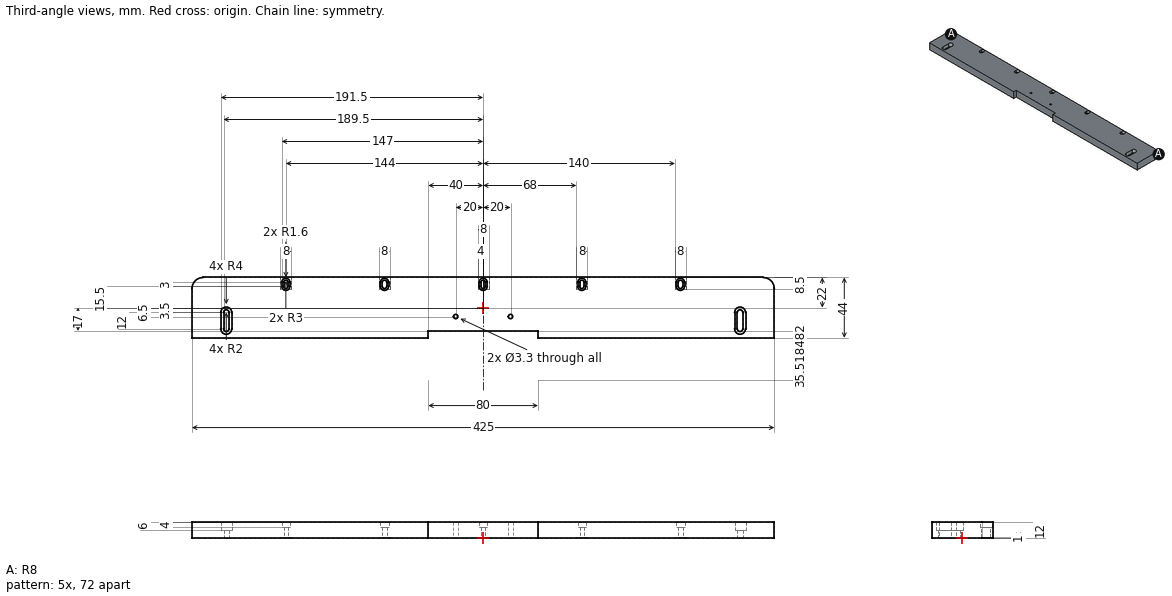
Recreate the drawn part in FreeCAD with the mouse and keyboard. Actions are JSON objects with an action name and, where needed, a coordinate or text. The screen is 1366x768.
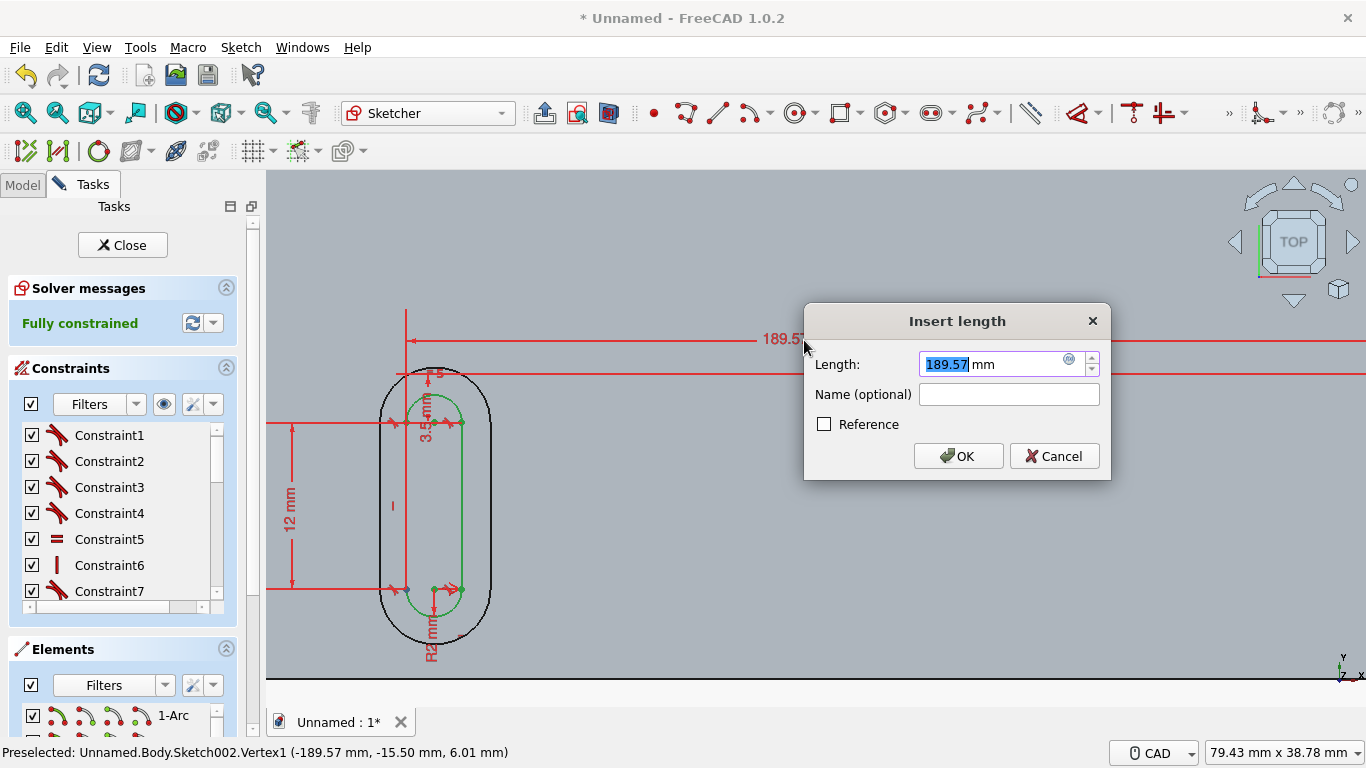
{"action": "type", "text": "189.5"}
{"action": "key", "text": "Return"}
{"action": "key", "text": "Escape"}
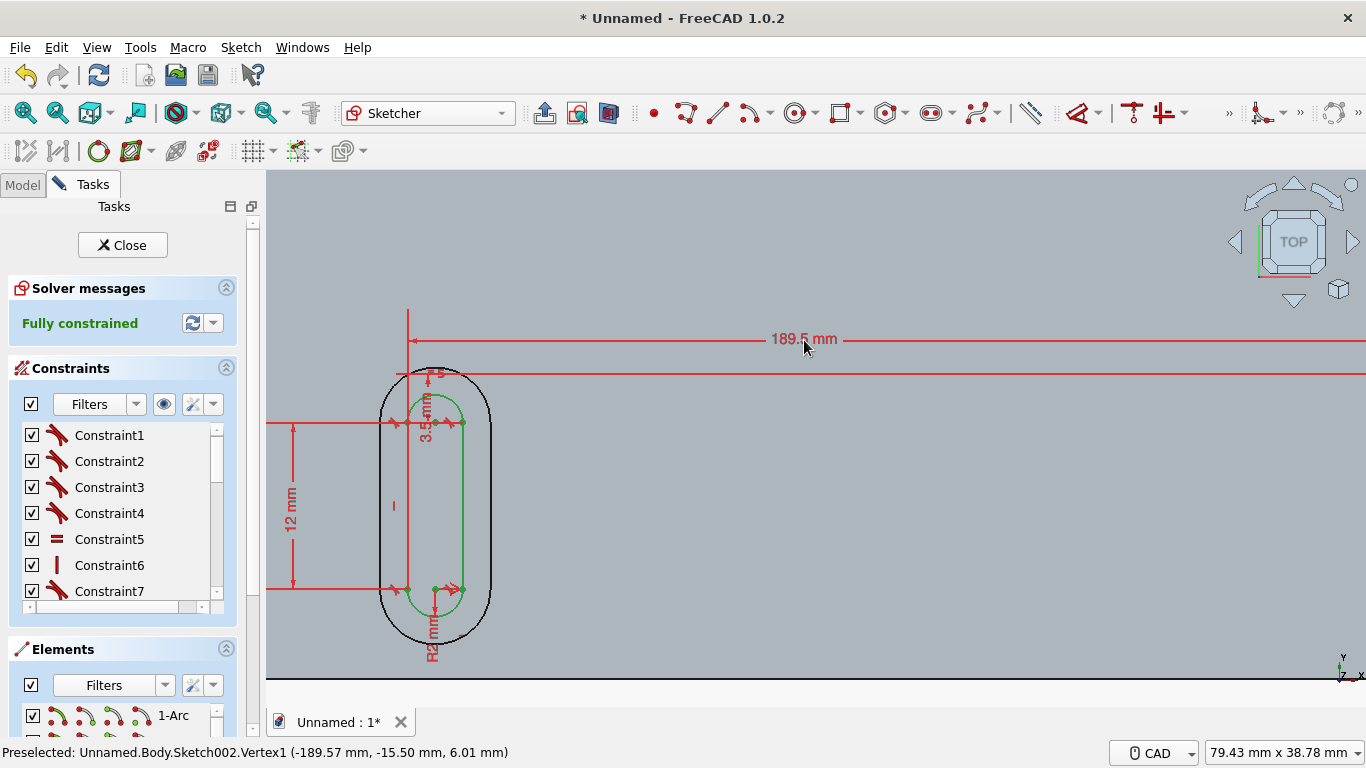
{"action": "left_click", "coordinate": [123, 245]}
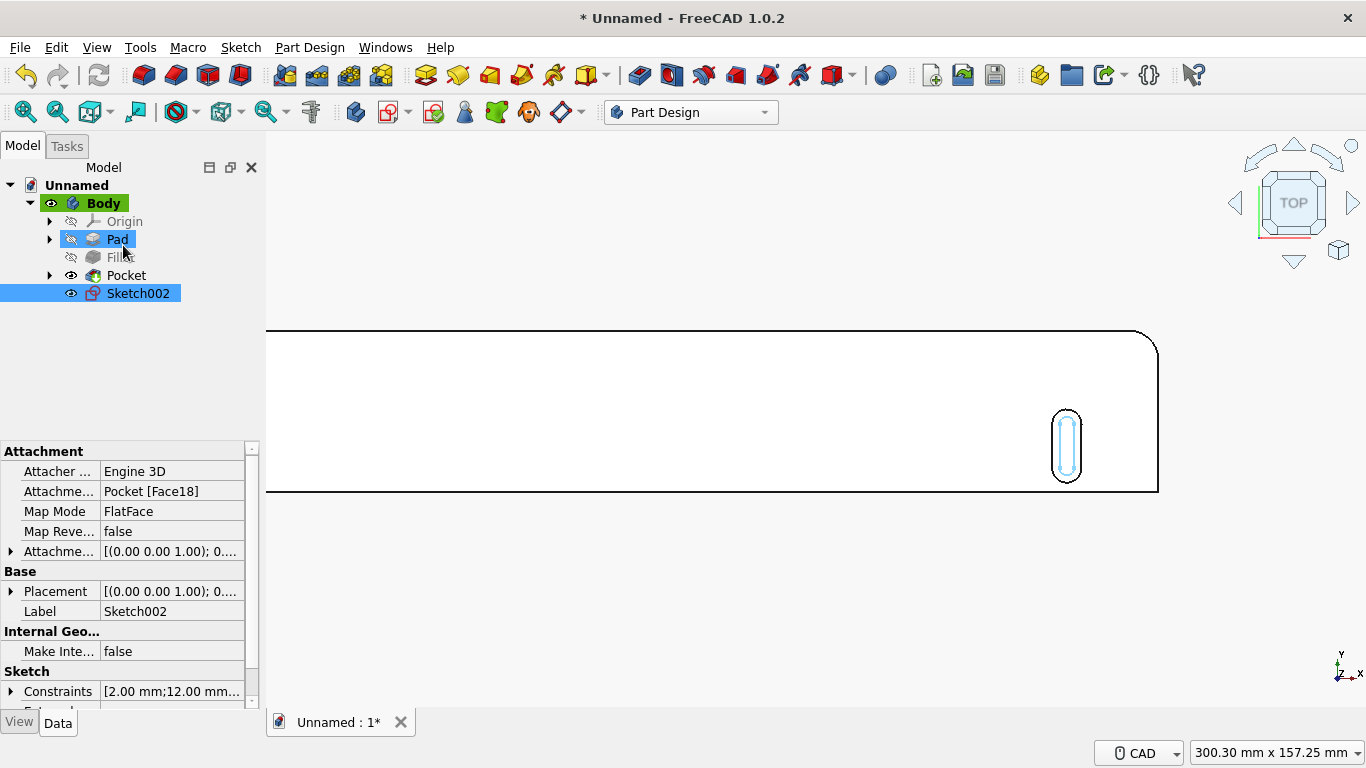
{"action": "left_click", "coordinate": [640, 76]}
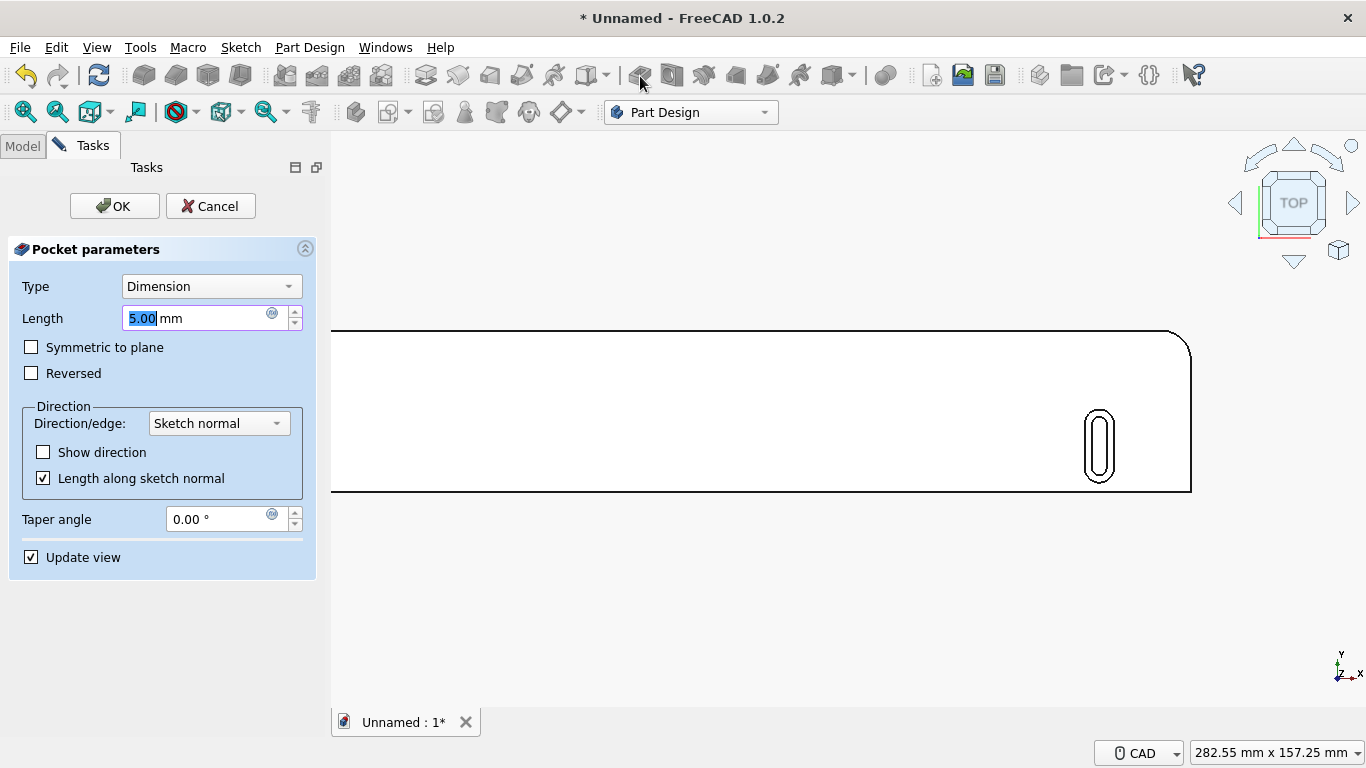
{"action": "left_click", "coordinate": [212, 286]}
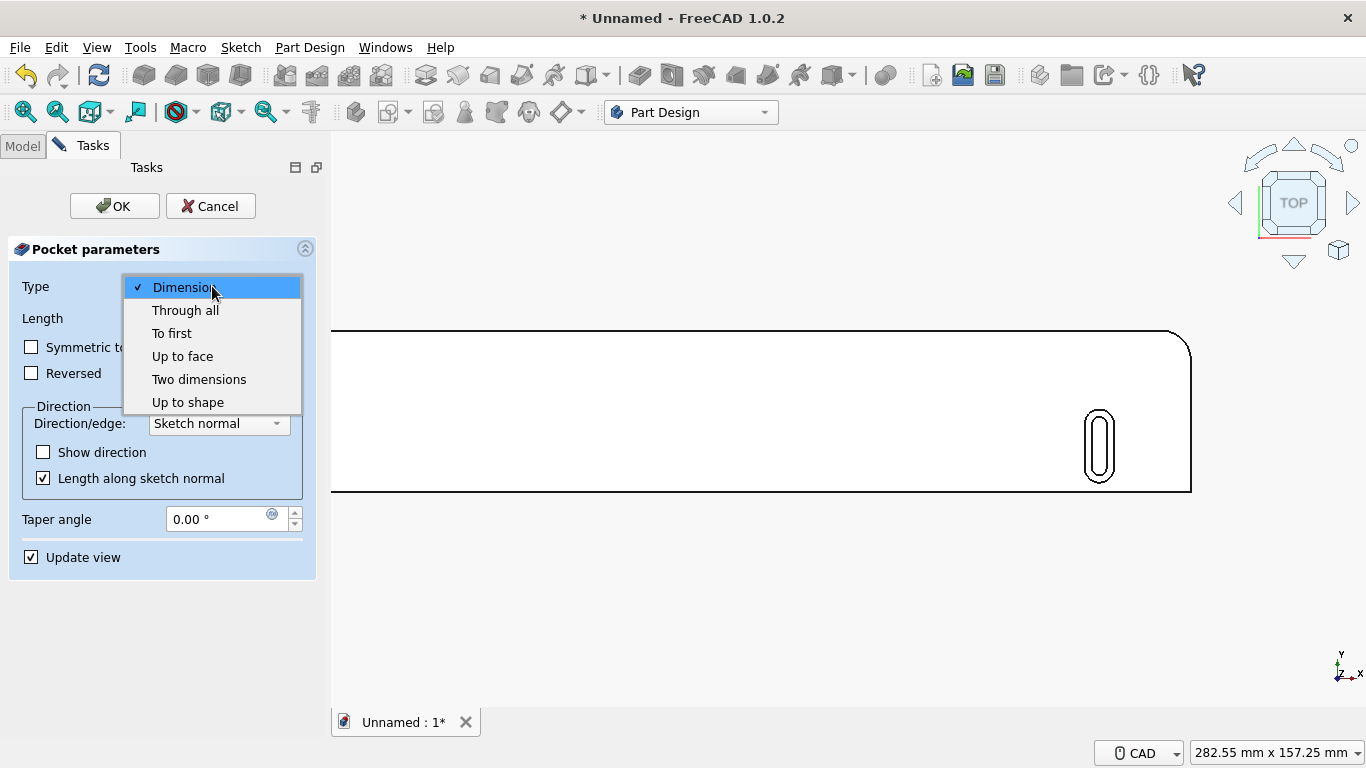
{"action": "left_click", "coordinate": [212, 310]}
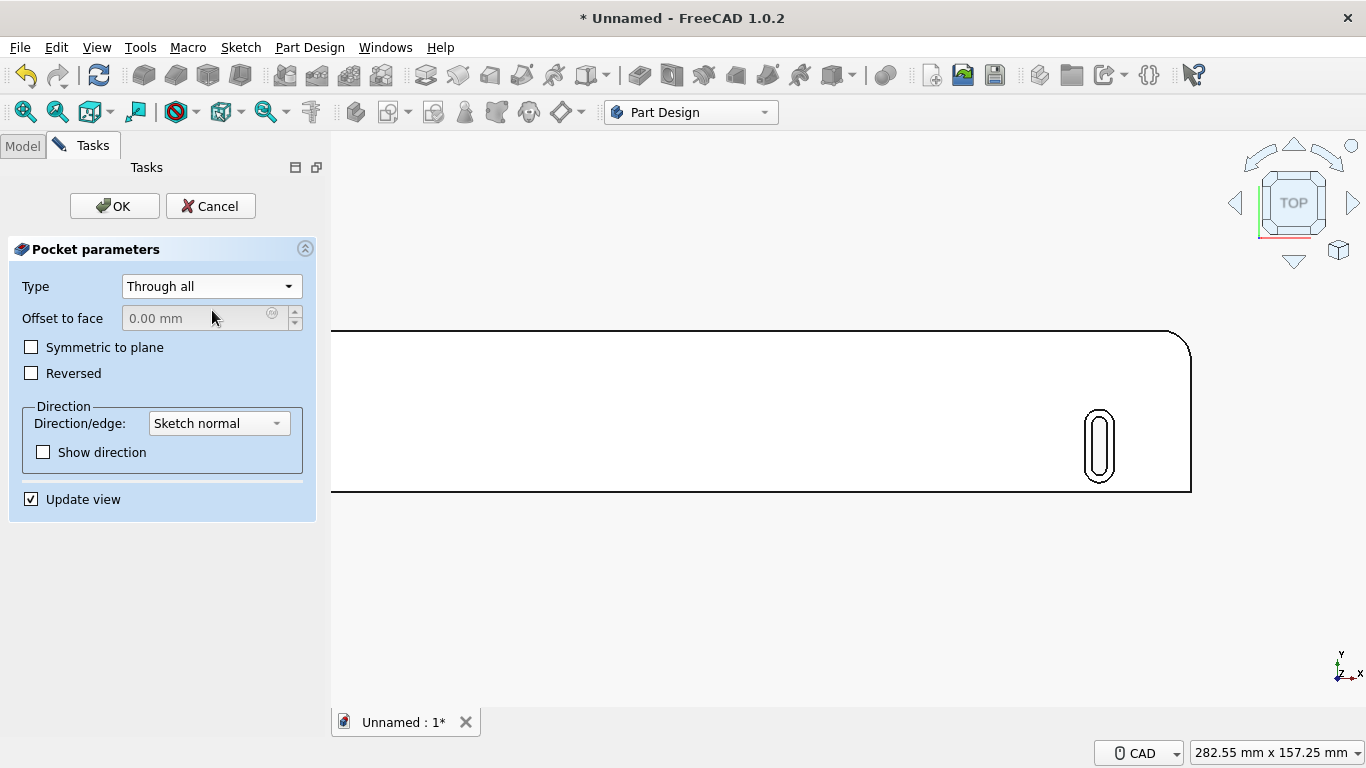
{"action": "left_click", "coordinate": [115, 206]}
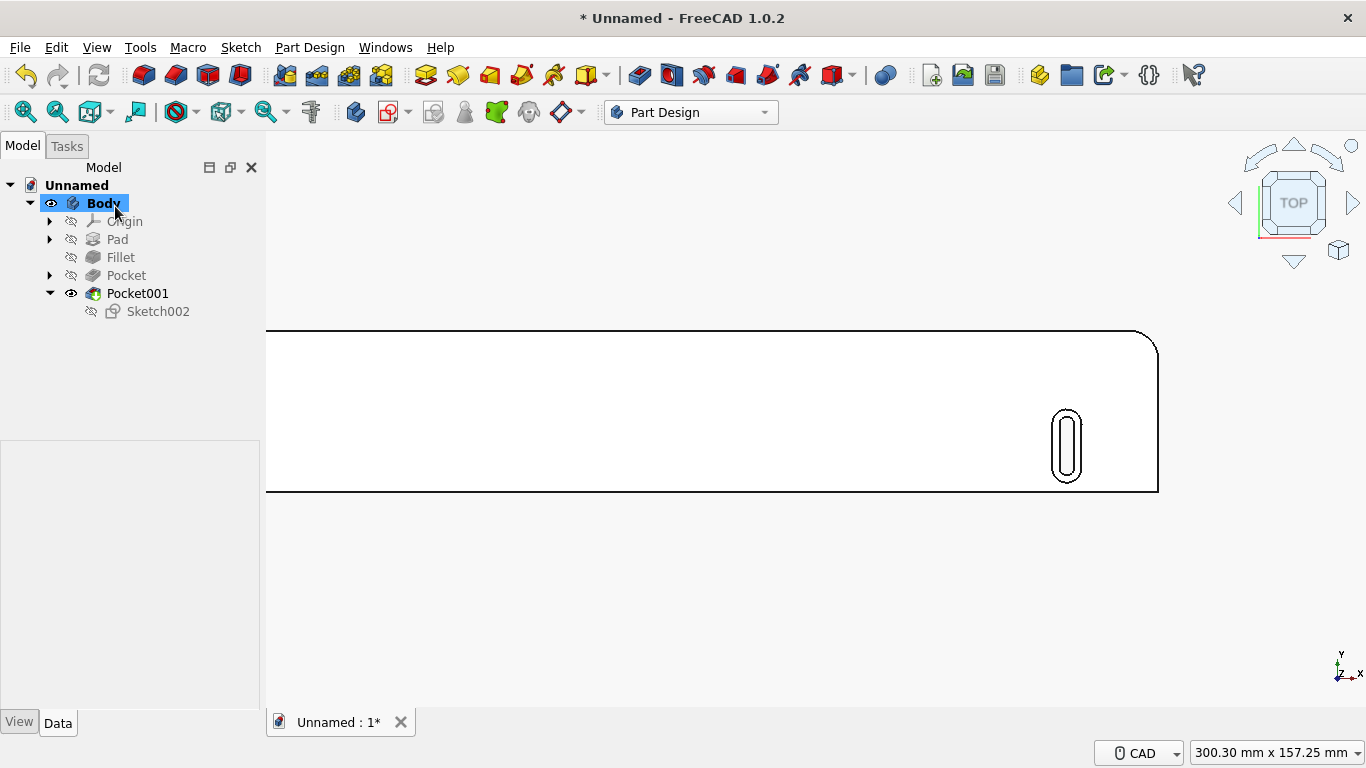
{"action": "left_click", "coordinate": [26, 112]}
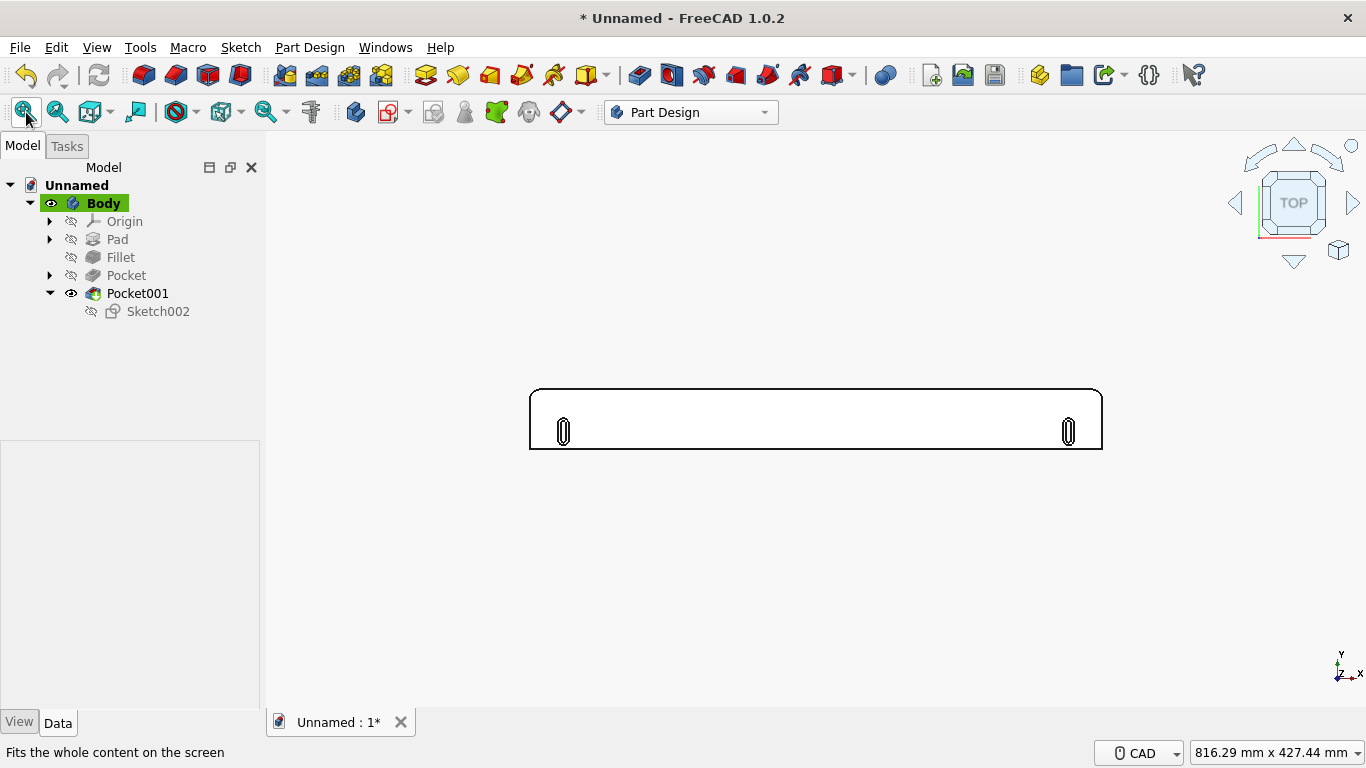
{"action": "left_click", "coordinate": [980, 418]}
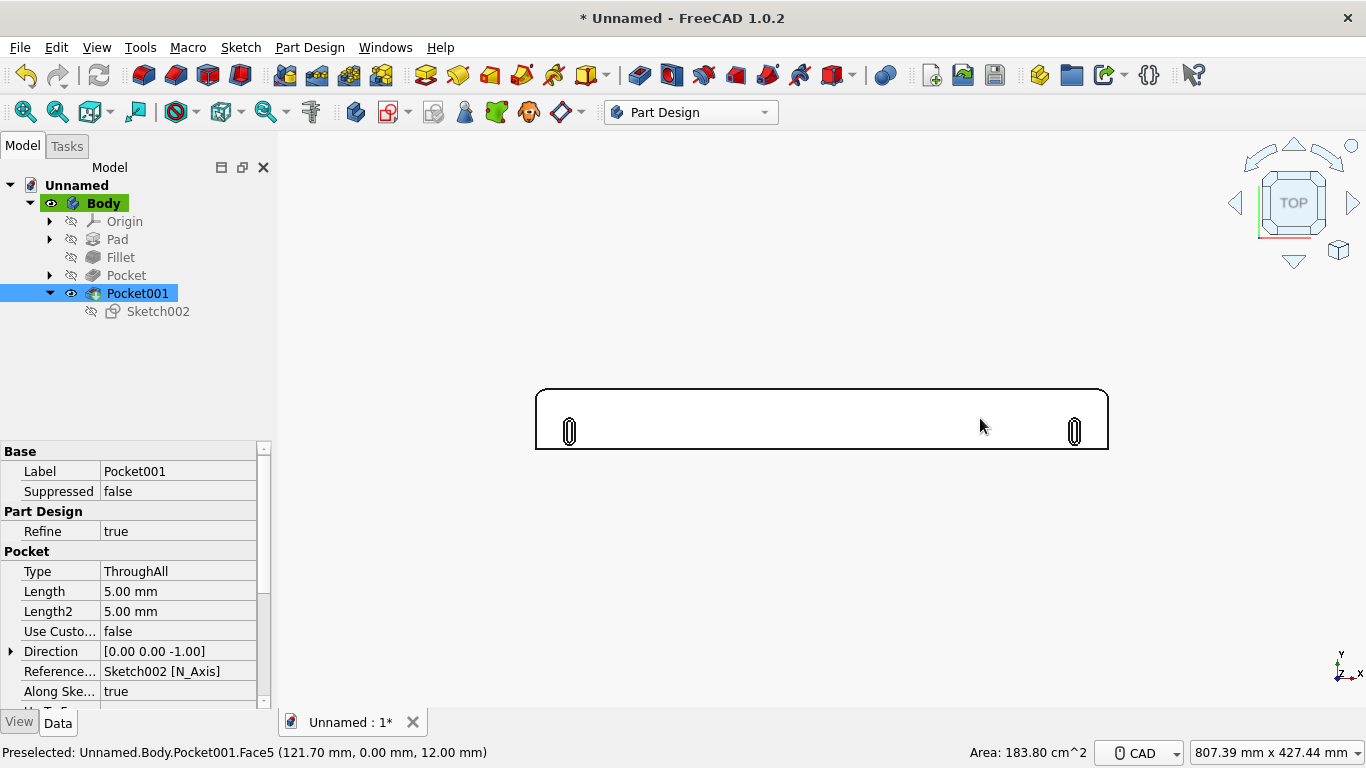
{"action": "left_click", "coordinate": [388, 112]}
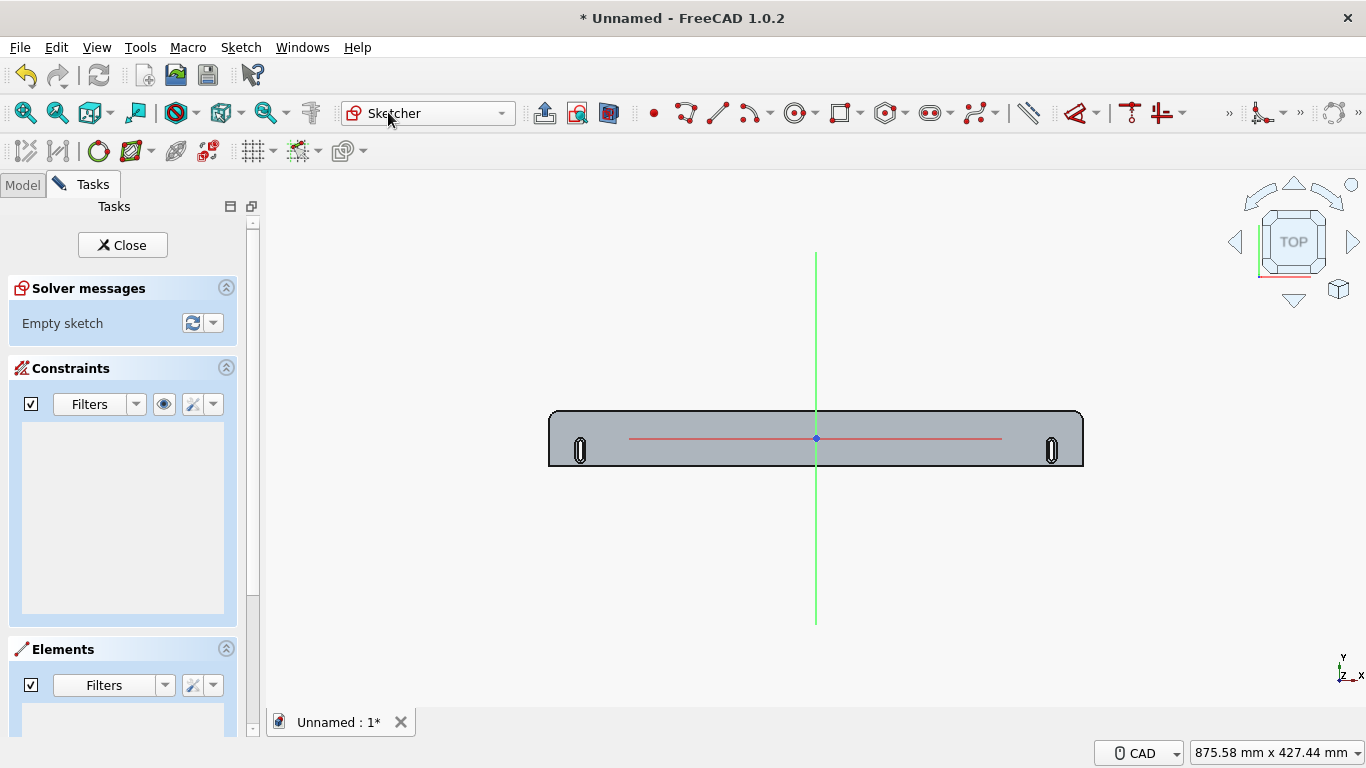
{"action": "scroll", "coordinate": [833, 480], "scroll_direction": "up", "scroll_amount": 8}